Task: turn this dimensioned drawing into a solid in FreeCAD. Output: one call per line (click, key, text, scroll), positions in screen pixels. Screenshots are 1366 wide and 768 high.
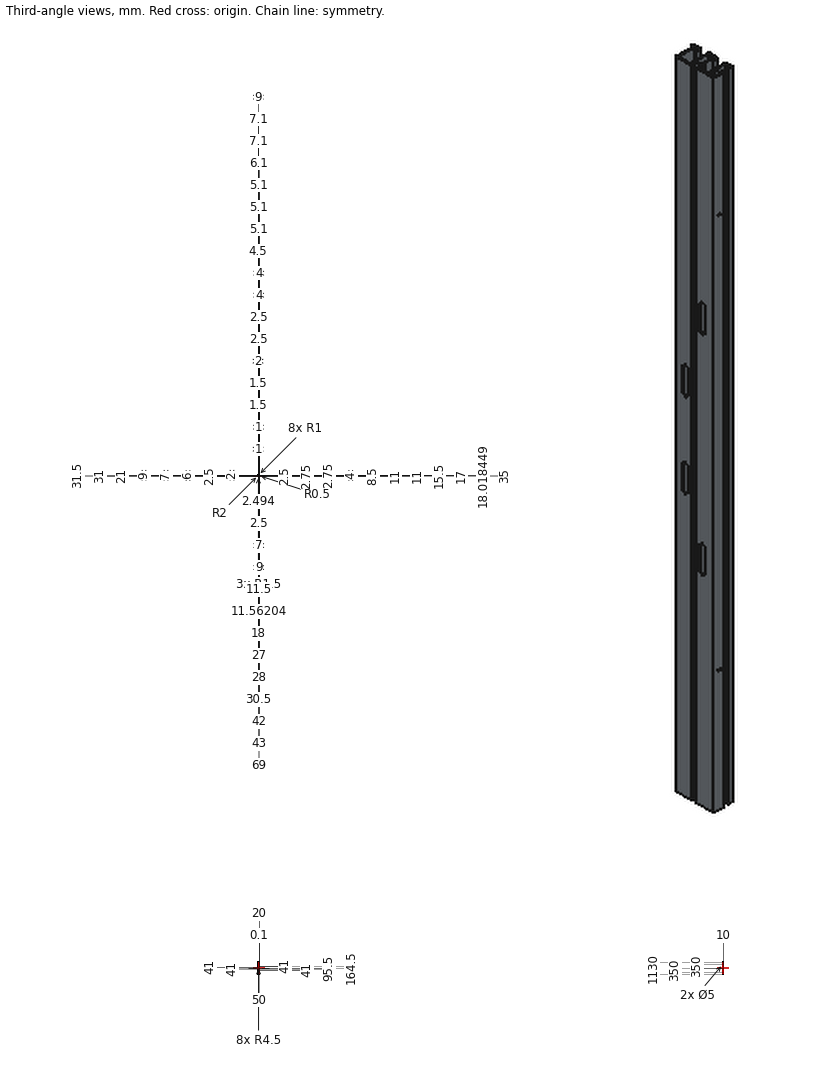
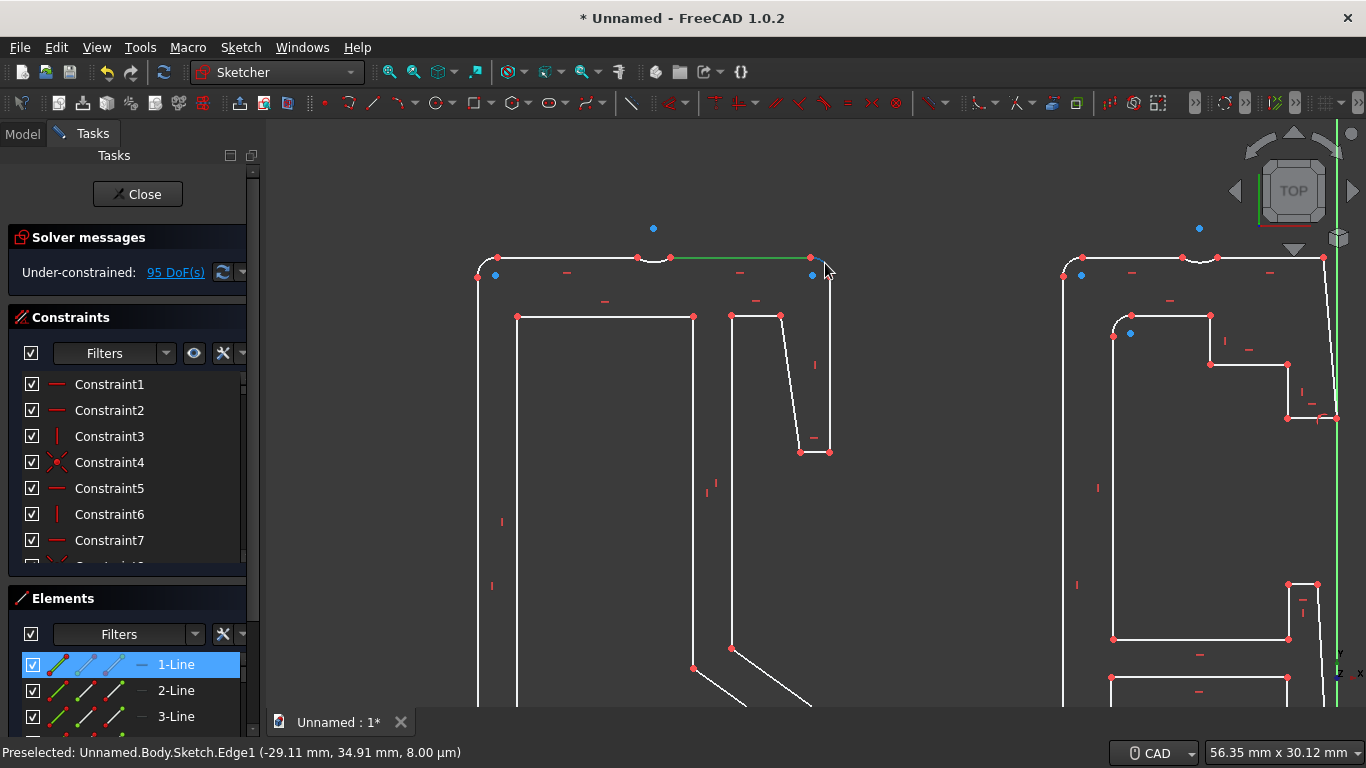
click(824, 263)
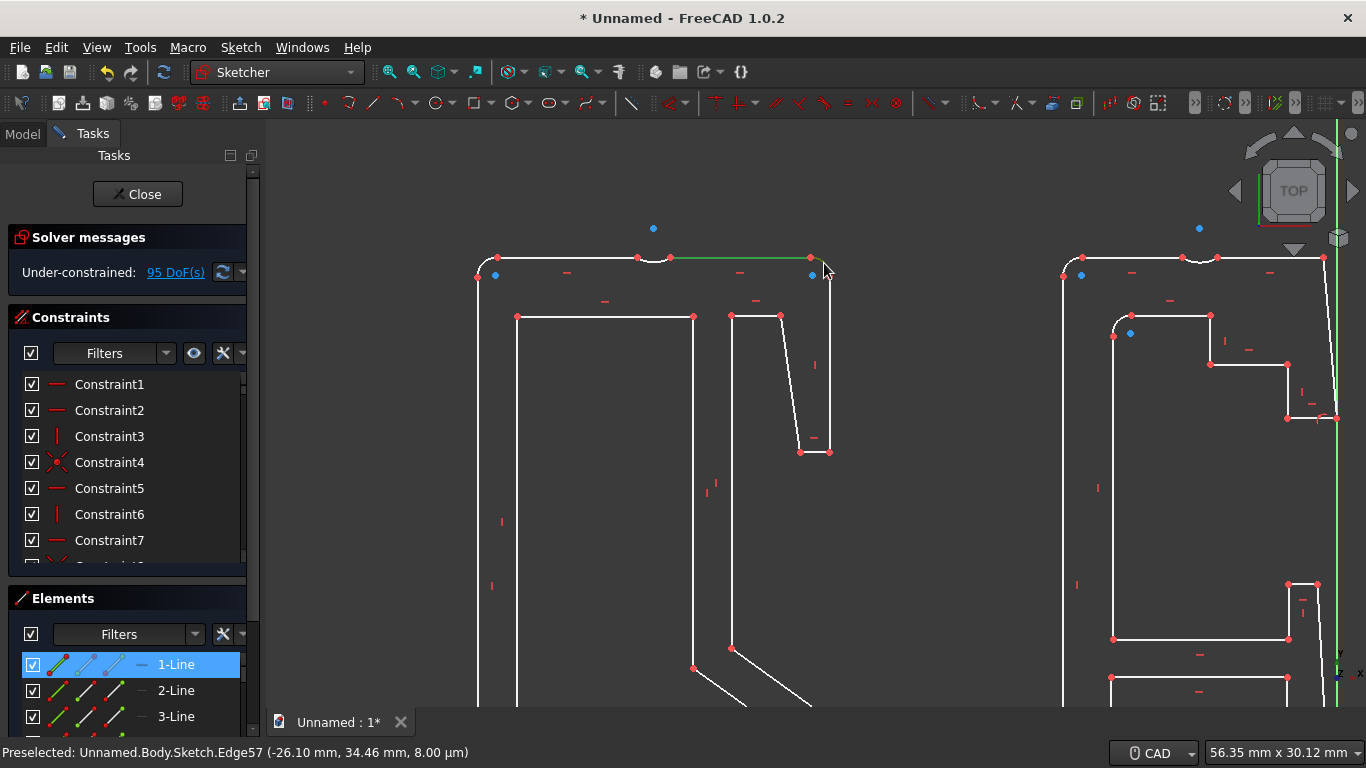
click(824, 104)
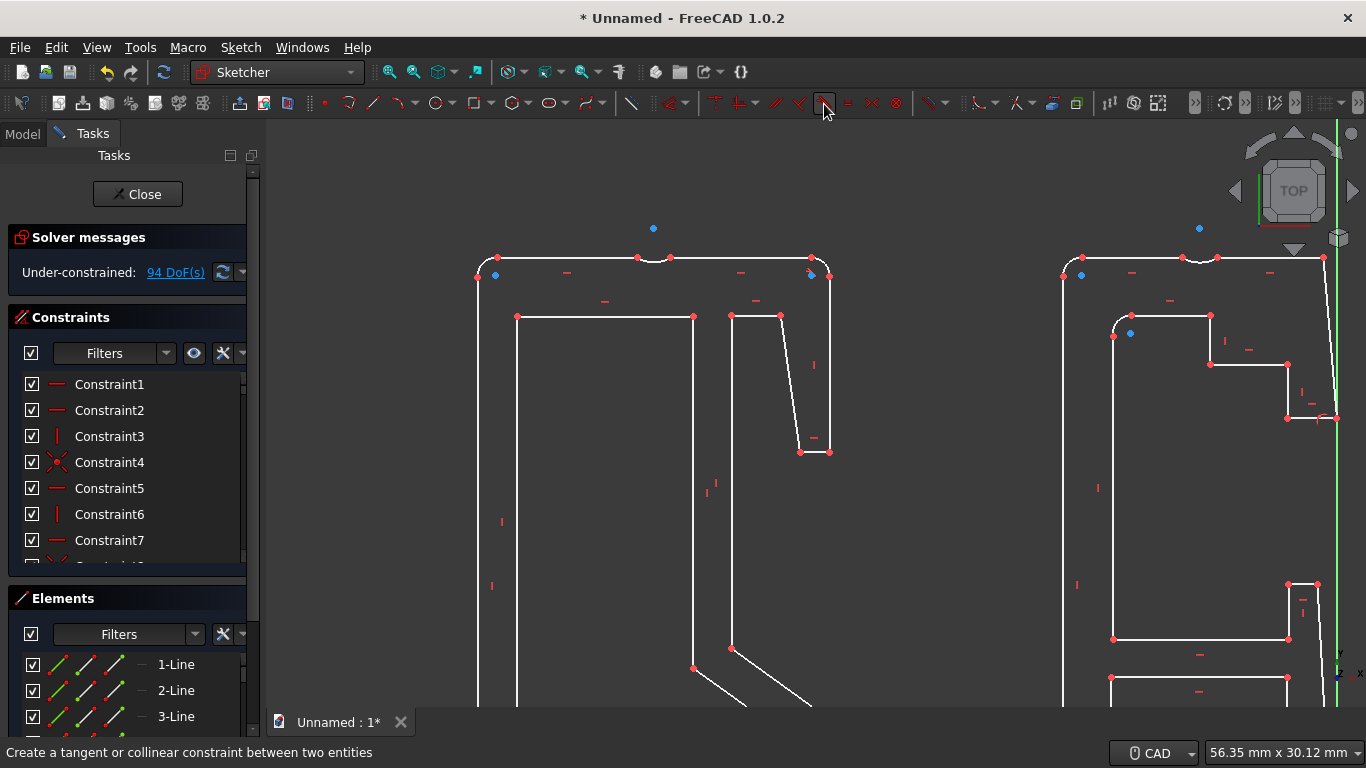
click(595, 258)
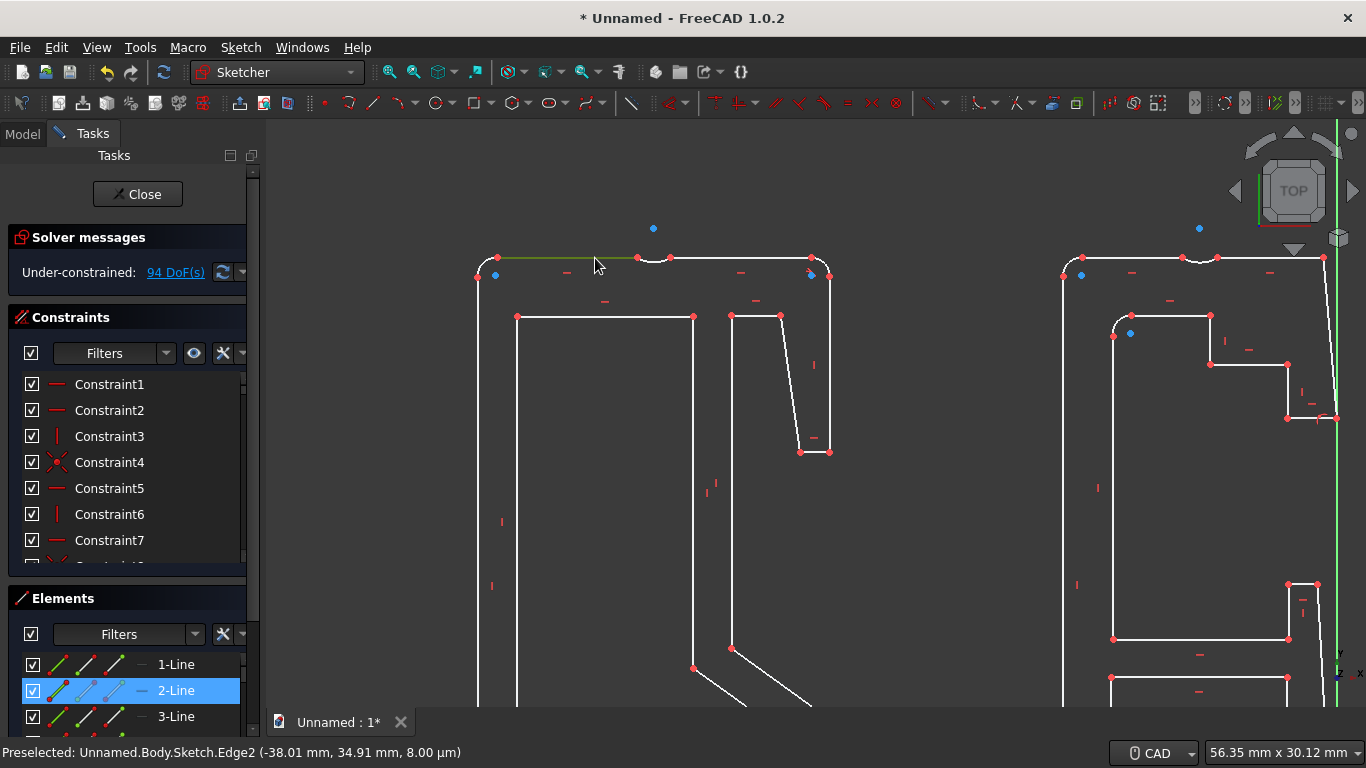
scroll(488, 259, up, 2)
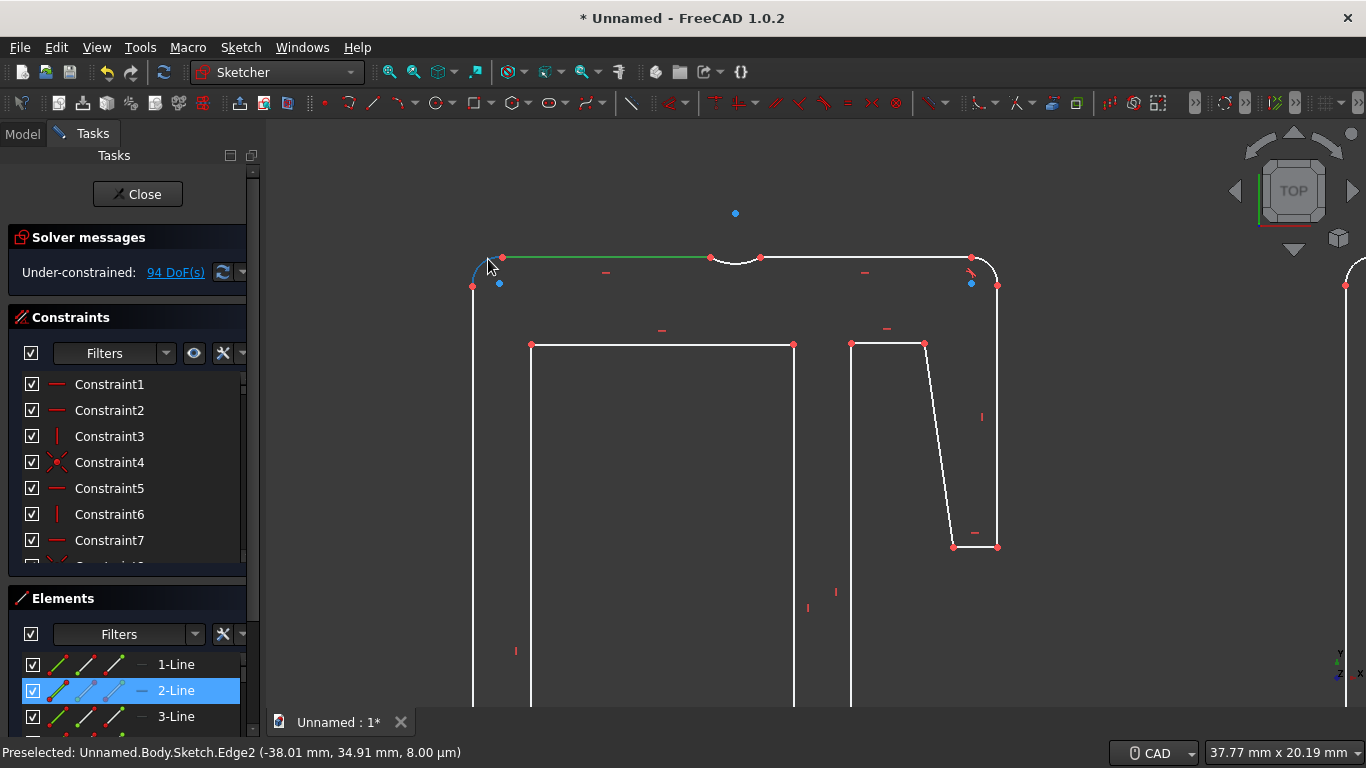
click(488, 260)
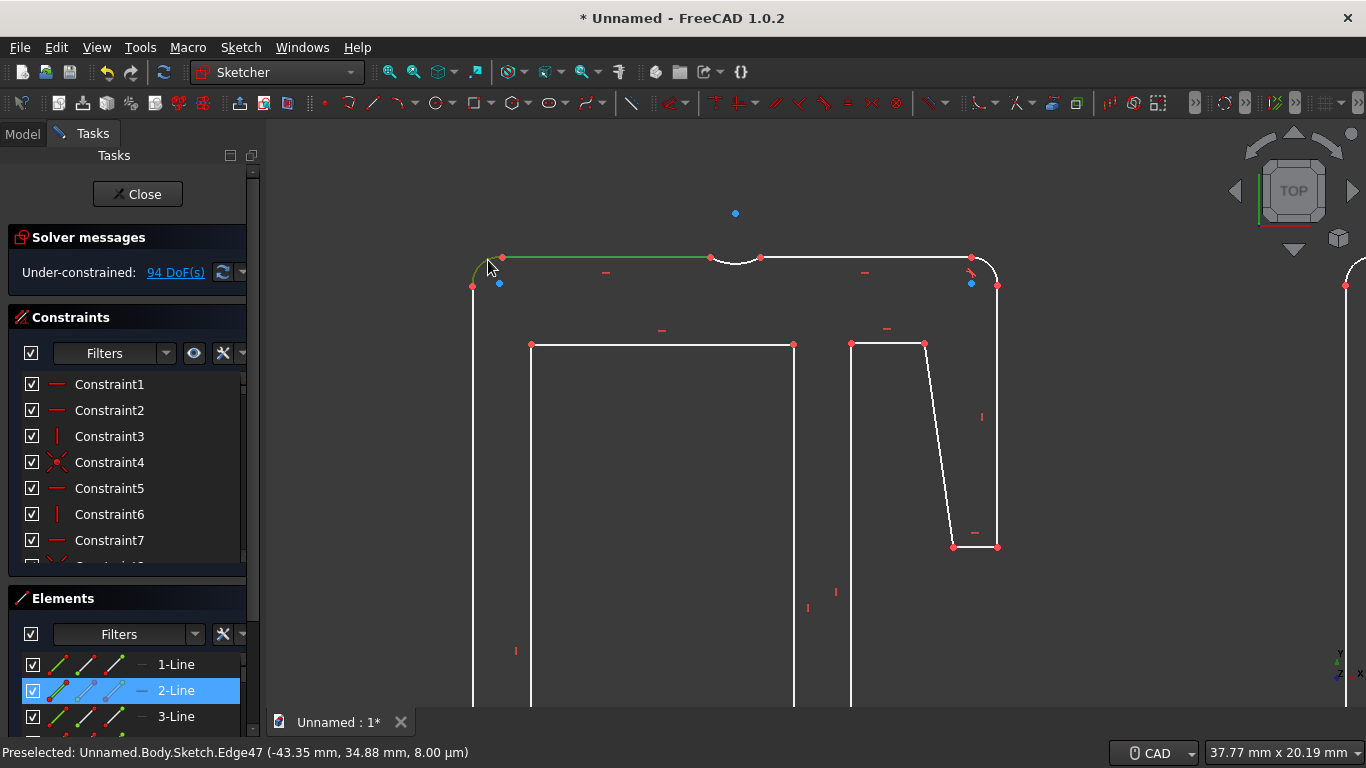
click(824, 104)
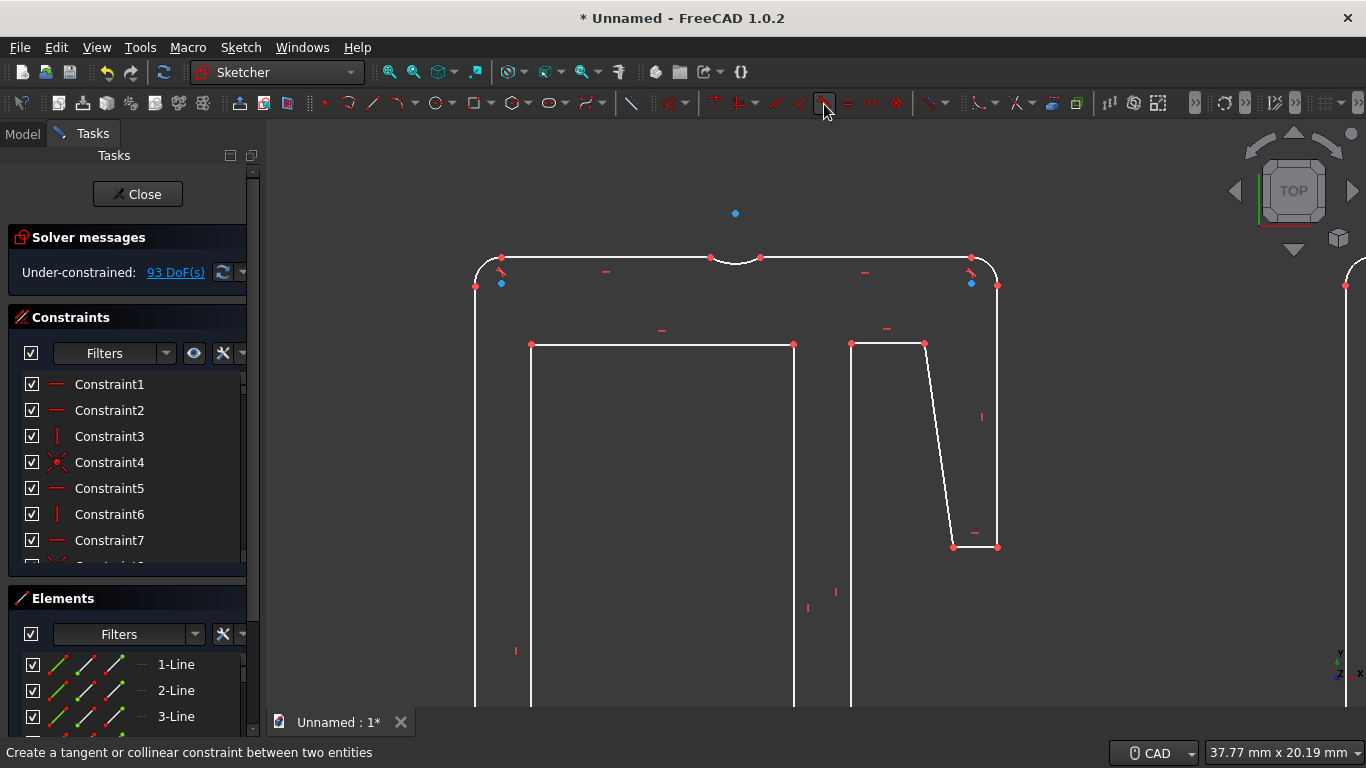
click(475, 562)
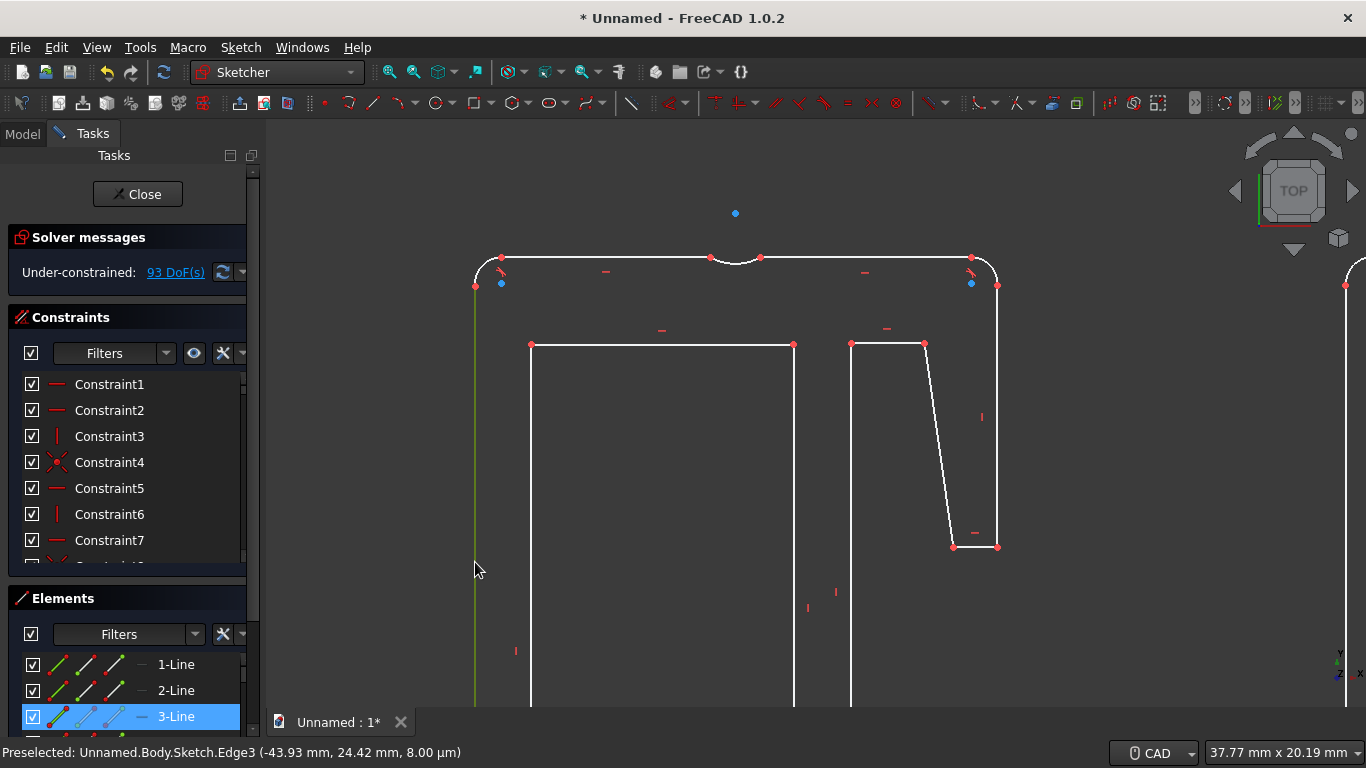
click(489, 261)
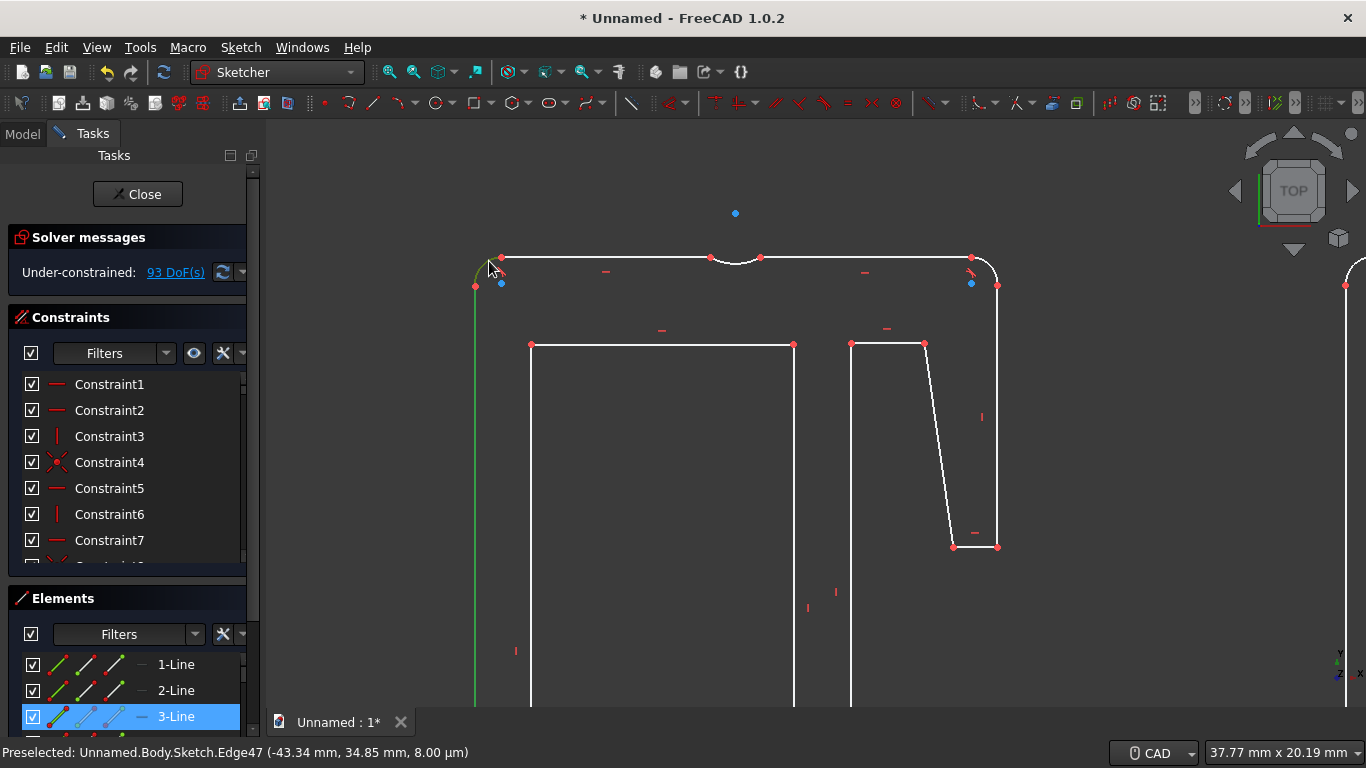
click(824, 104)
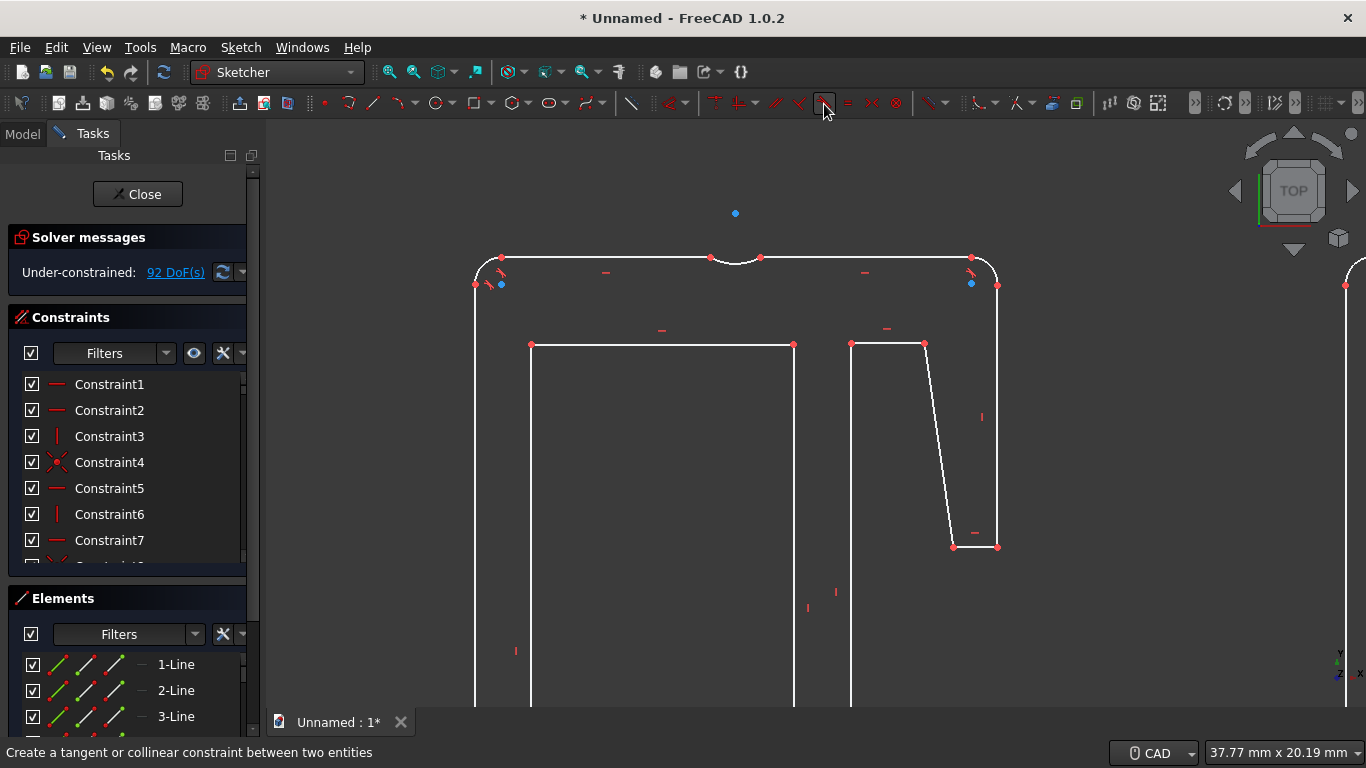
scroll(753, 262, down, 6)